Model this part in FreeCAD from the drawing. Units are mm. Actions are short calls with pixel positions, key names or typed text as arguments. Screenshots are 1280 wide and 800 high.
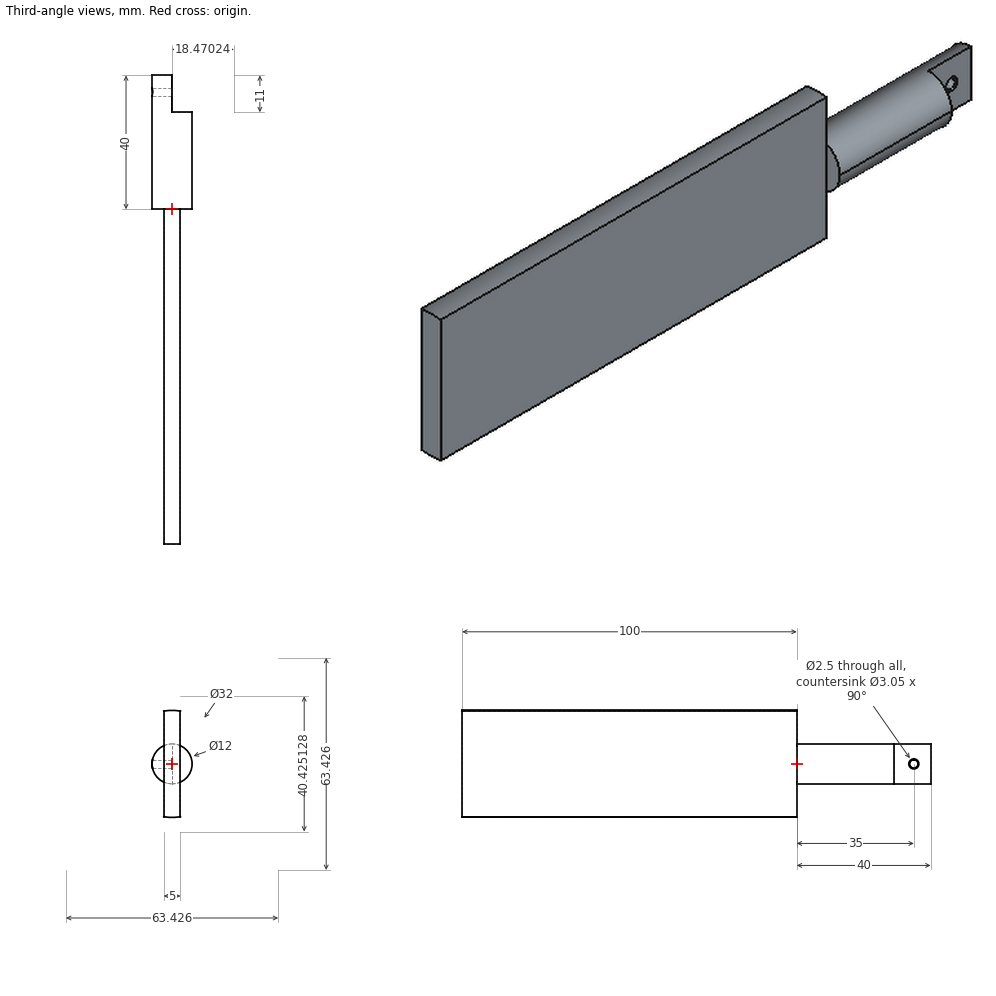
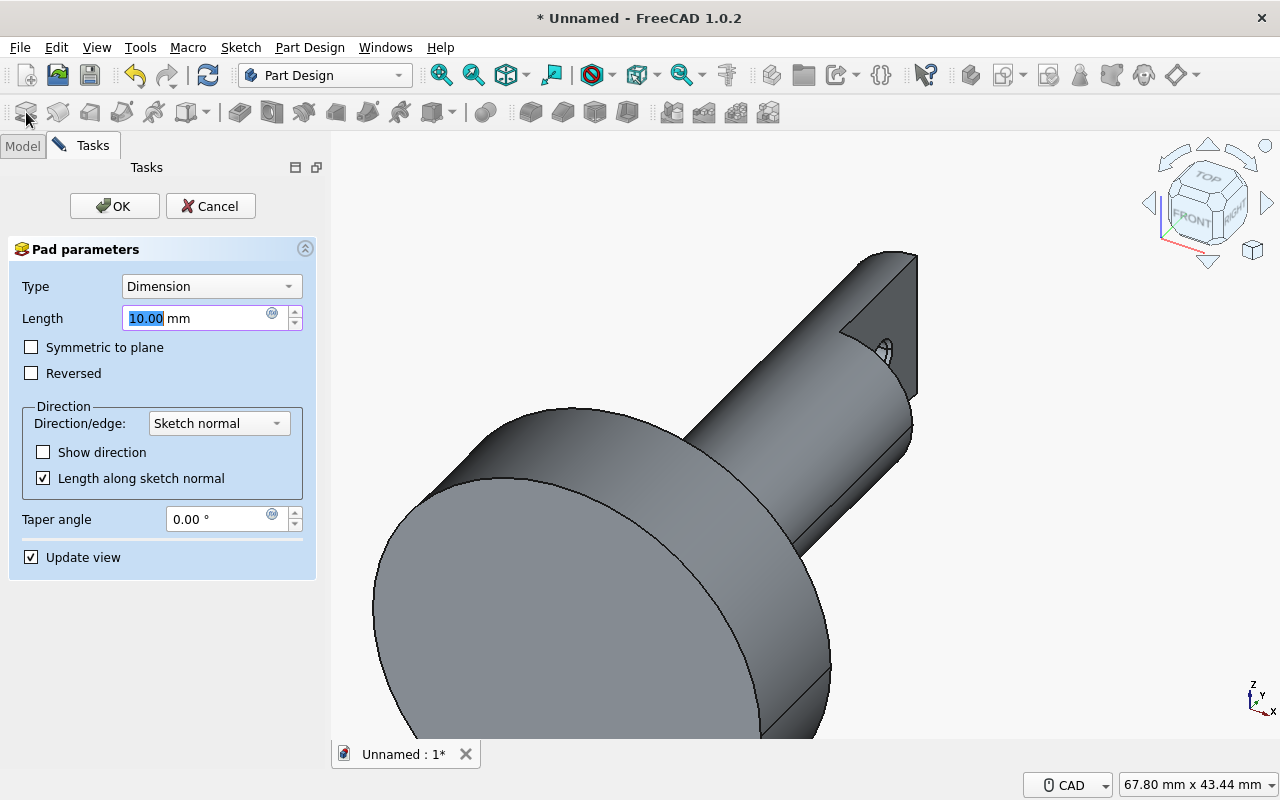
text(100)
key(Tab)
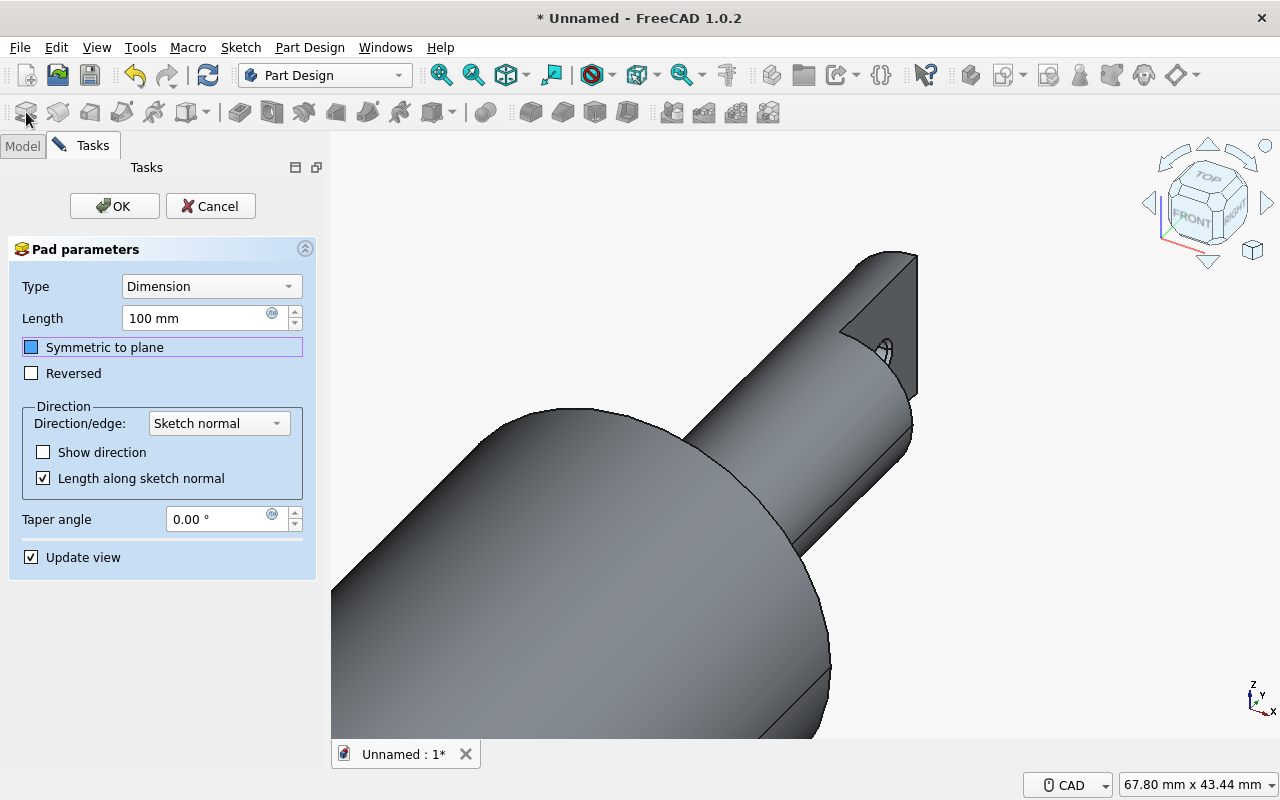
click(115, 206)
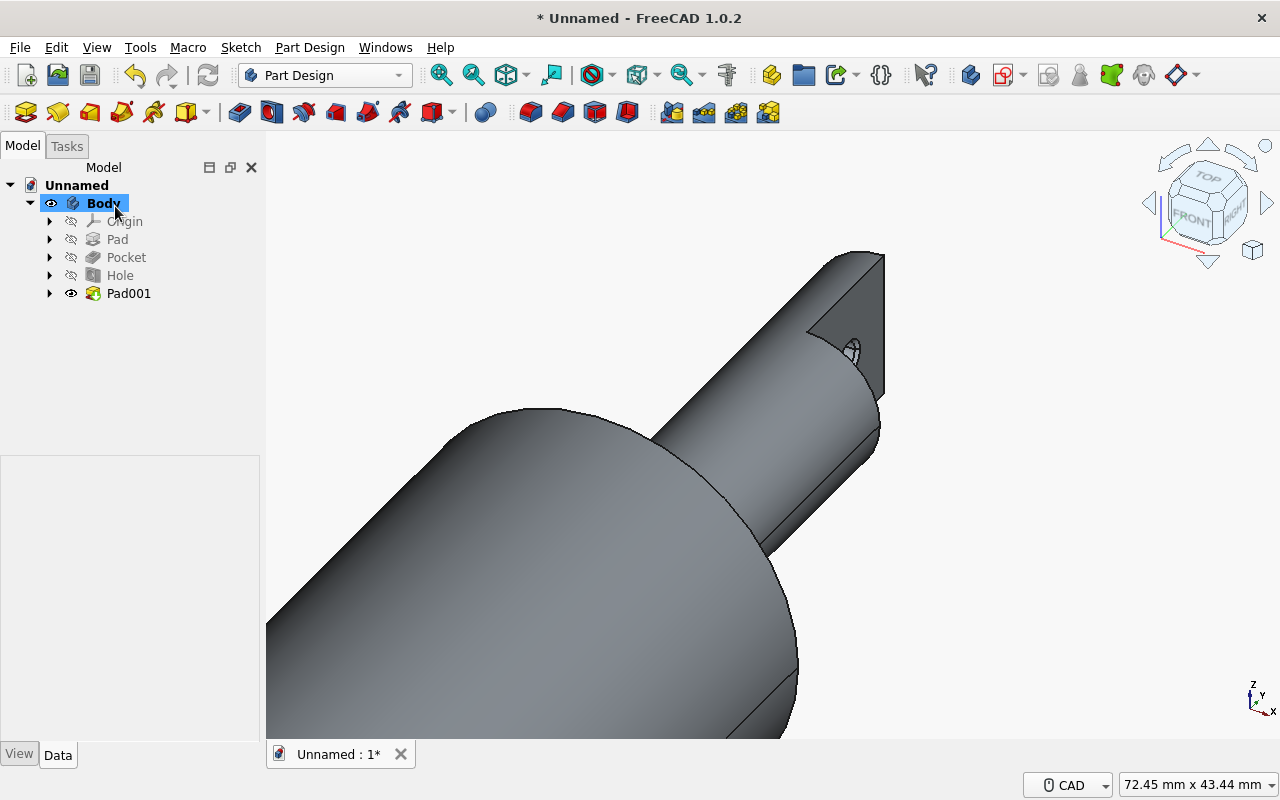
click(442, 76)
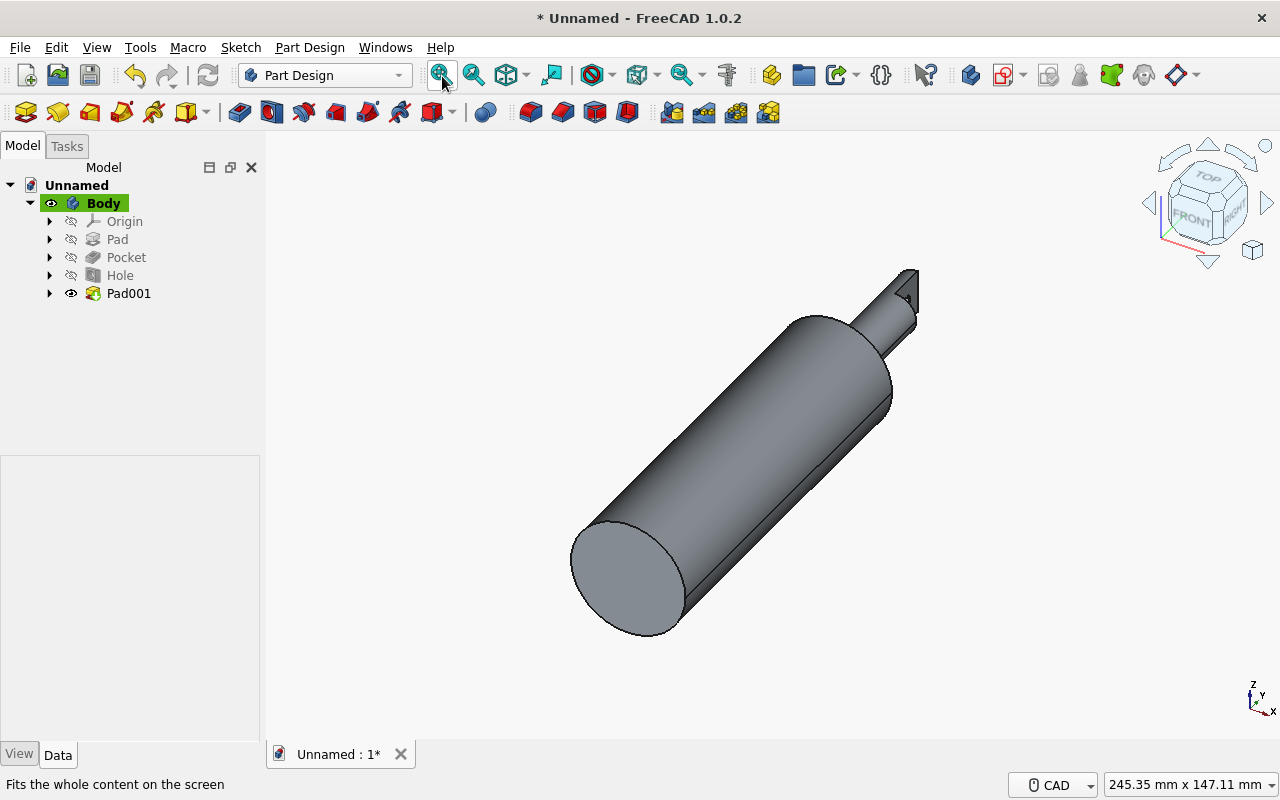
click(628, 578)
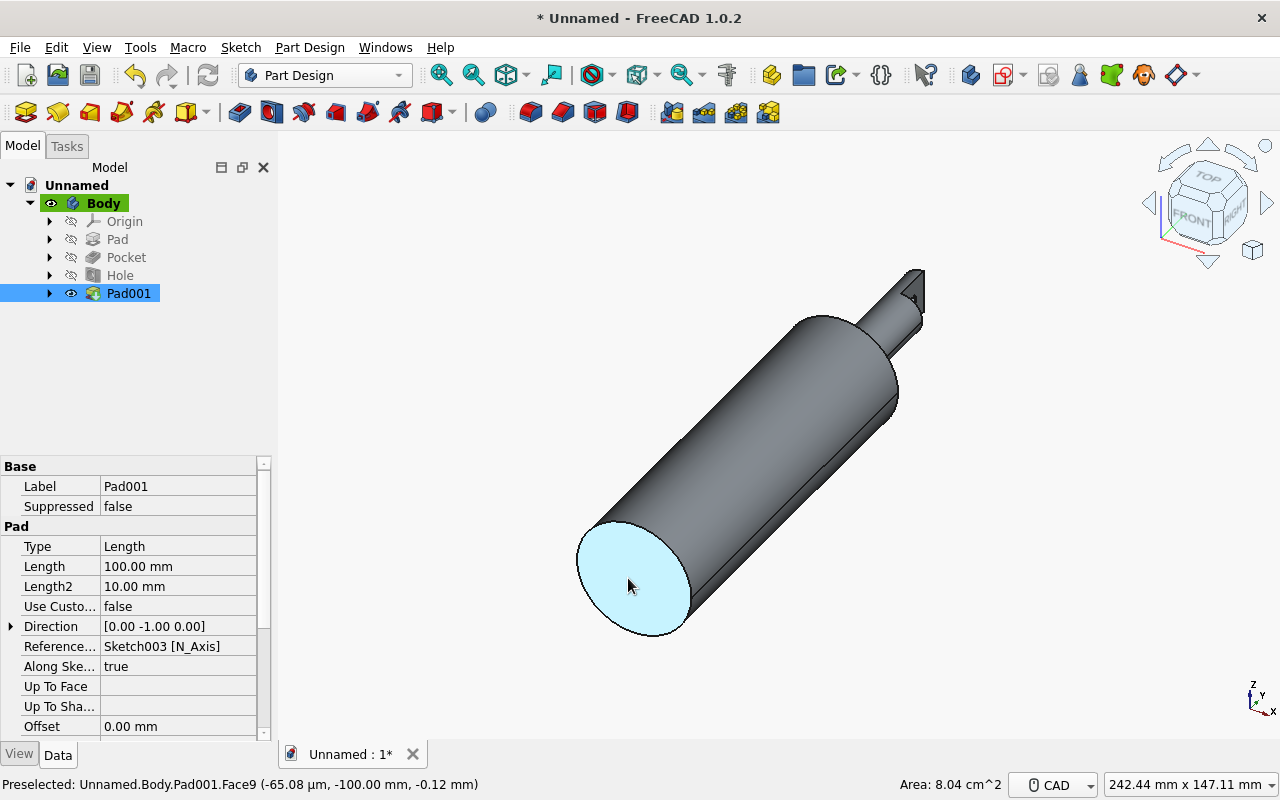
click(1004, 76)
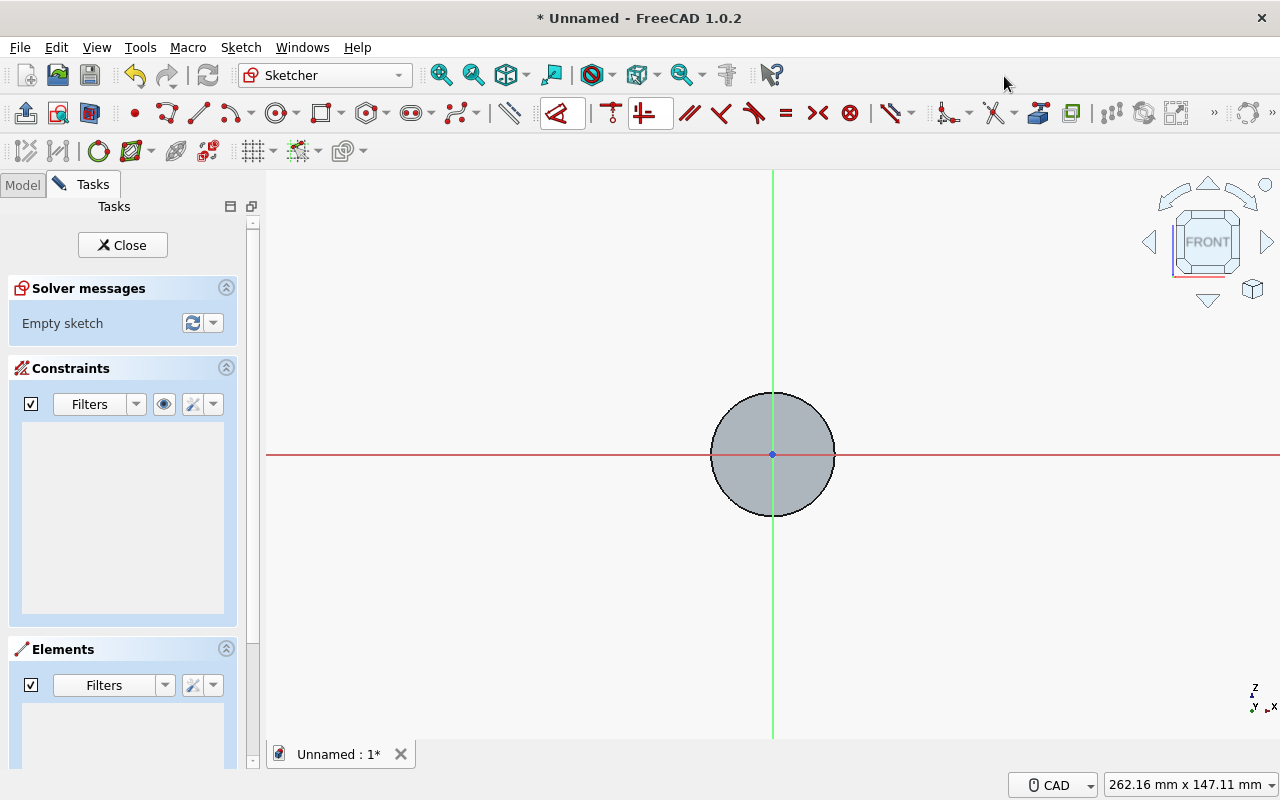
scroll(912, 454, up, 2)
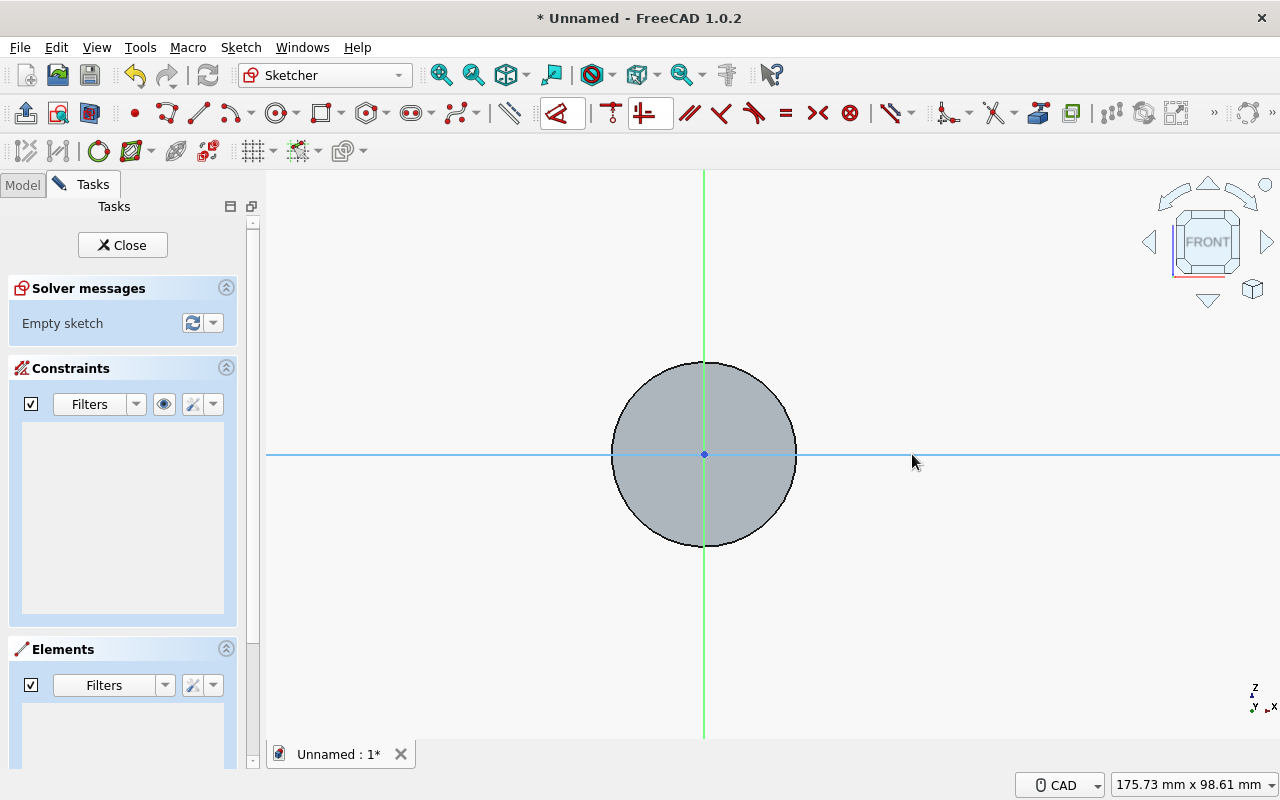
click(344, 114)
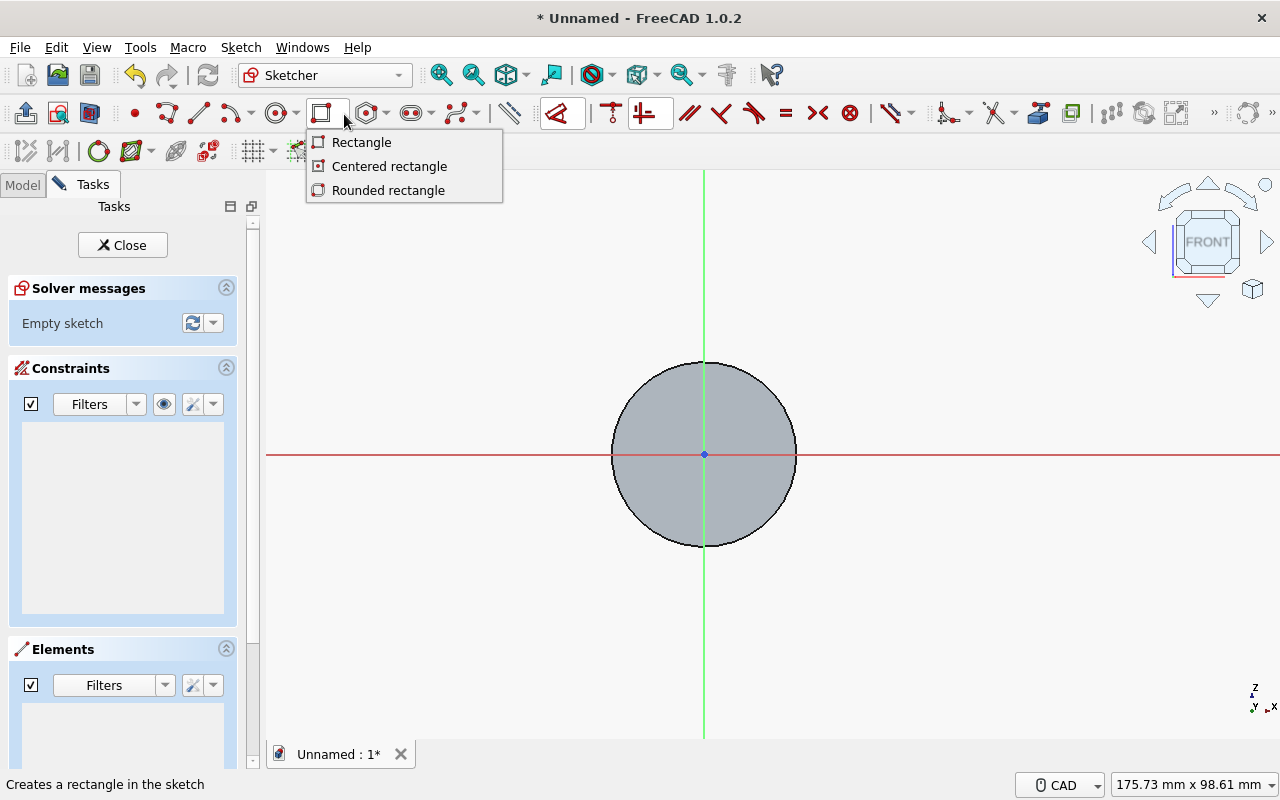
click(404, 166)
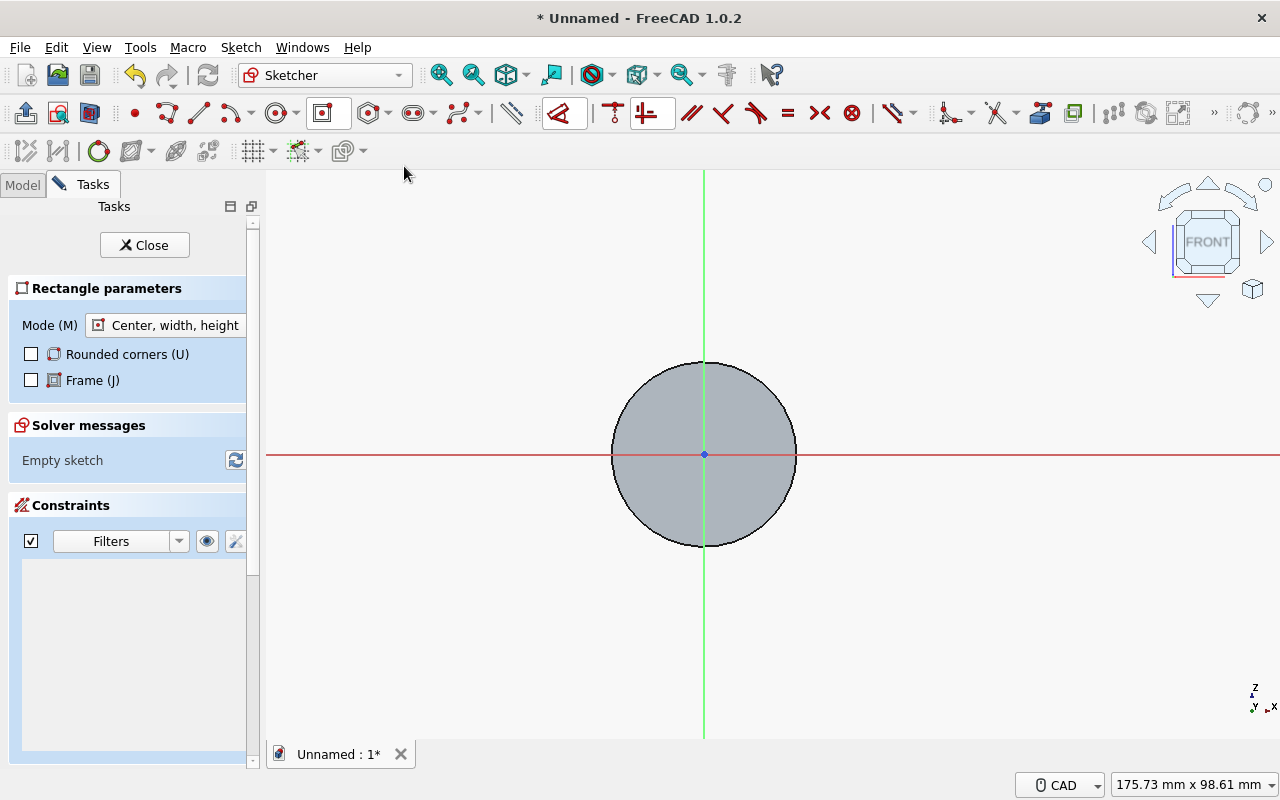
click(704, 454)
move(887, 272)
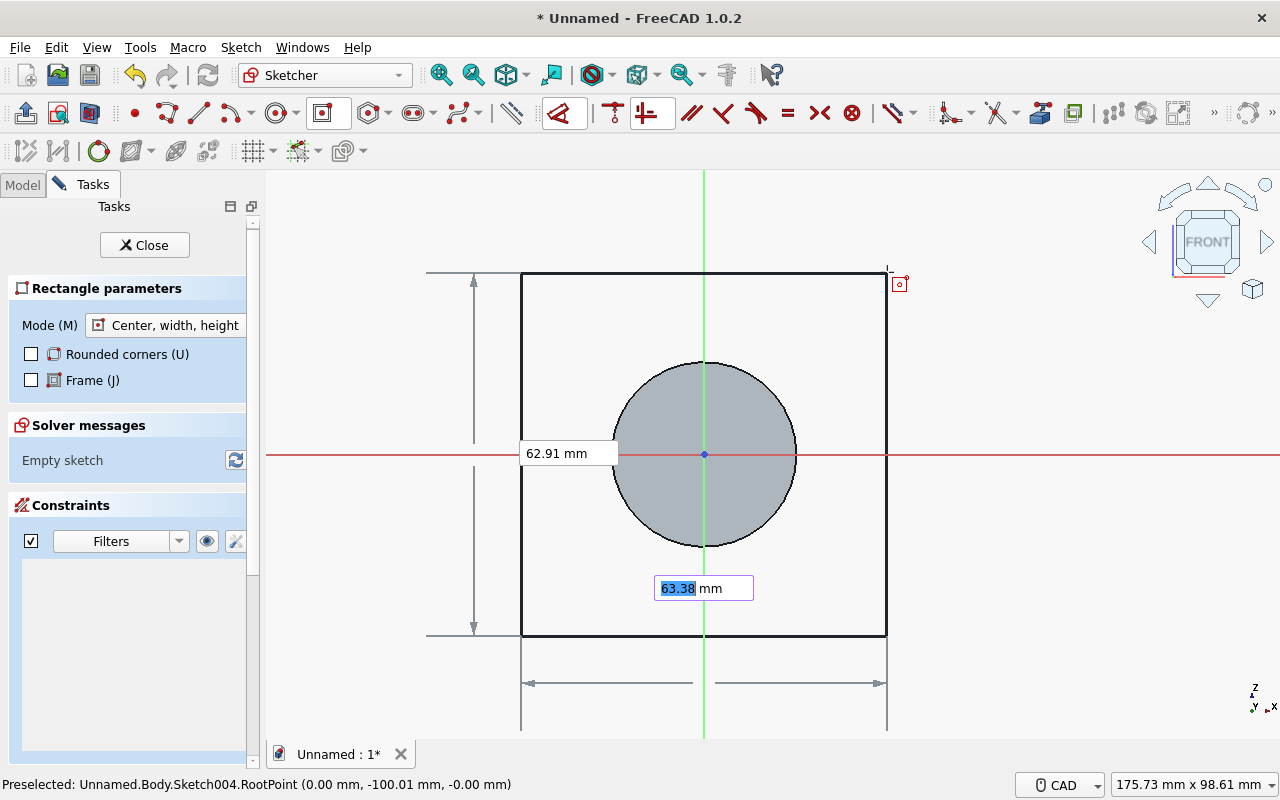
text(63.426)
key(Tab)
text(63.426)
key(Return)